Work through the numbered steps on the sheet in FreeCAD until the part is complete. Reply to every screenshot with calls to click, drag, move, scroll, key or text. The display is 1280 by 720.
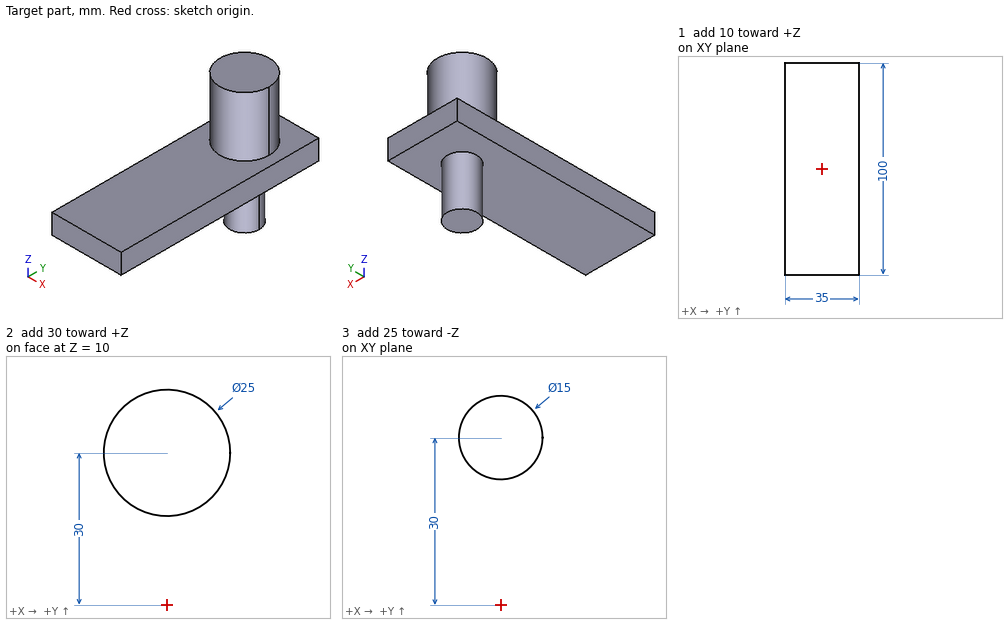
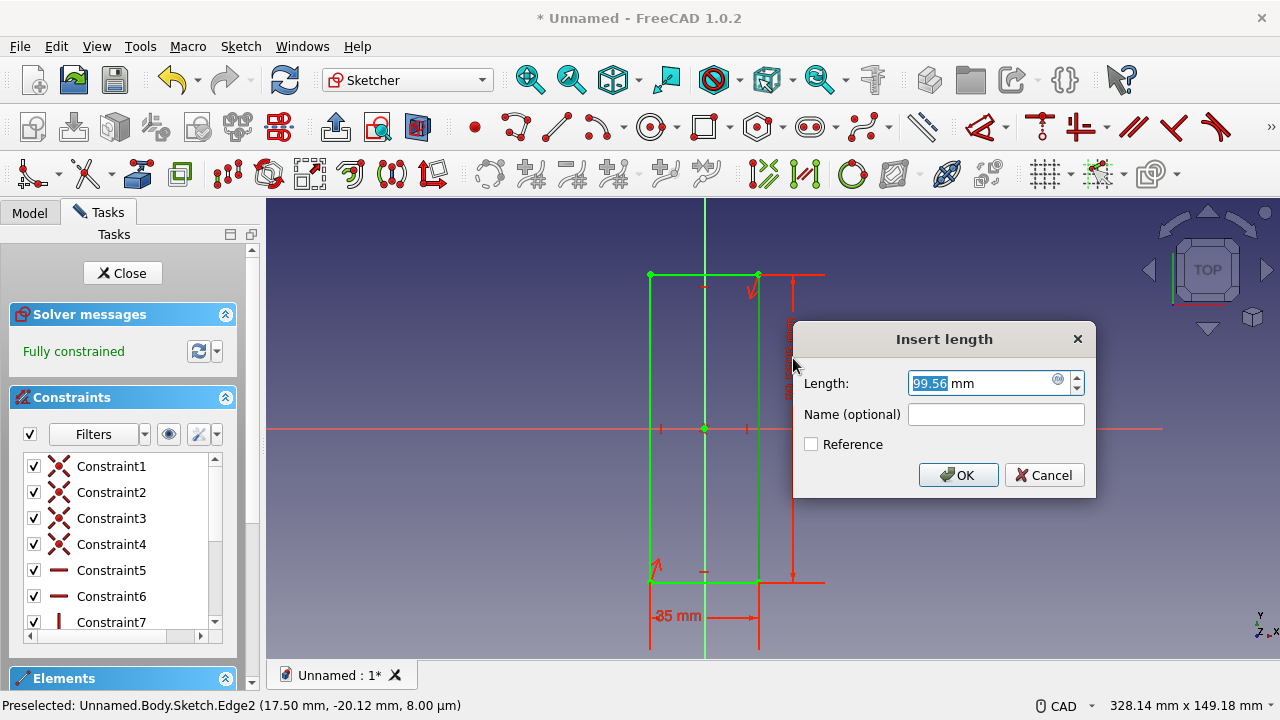
text(100)
key(Return)
key(Escape)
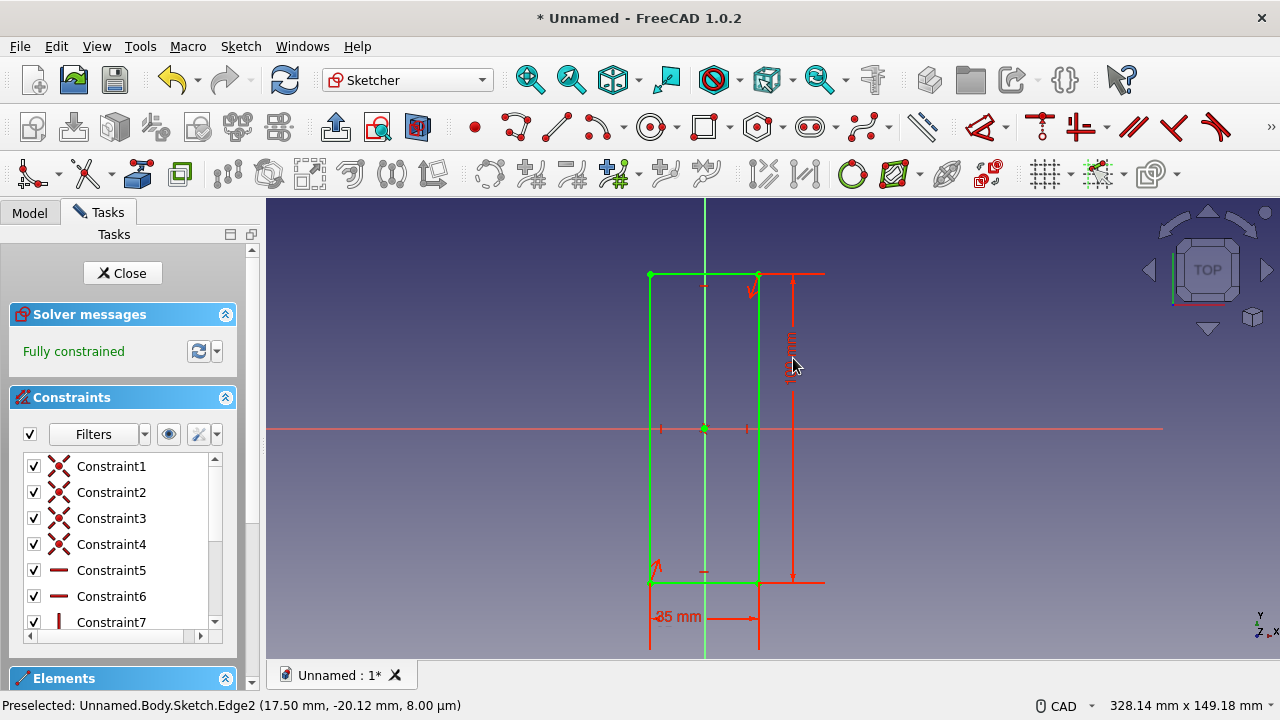
click(123, 273)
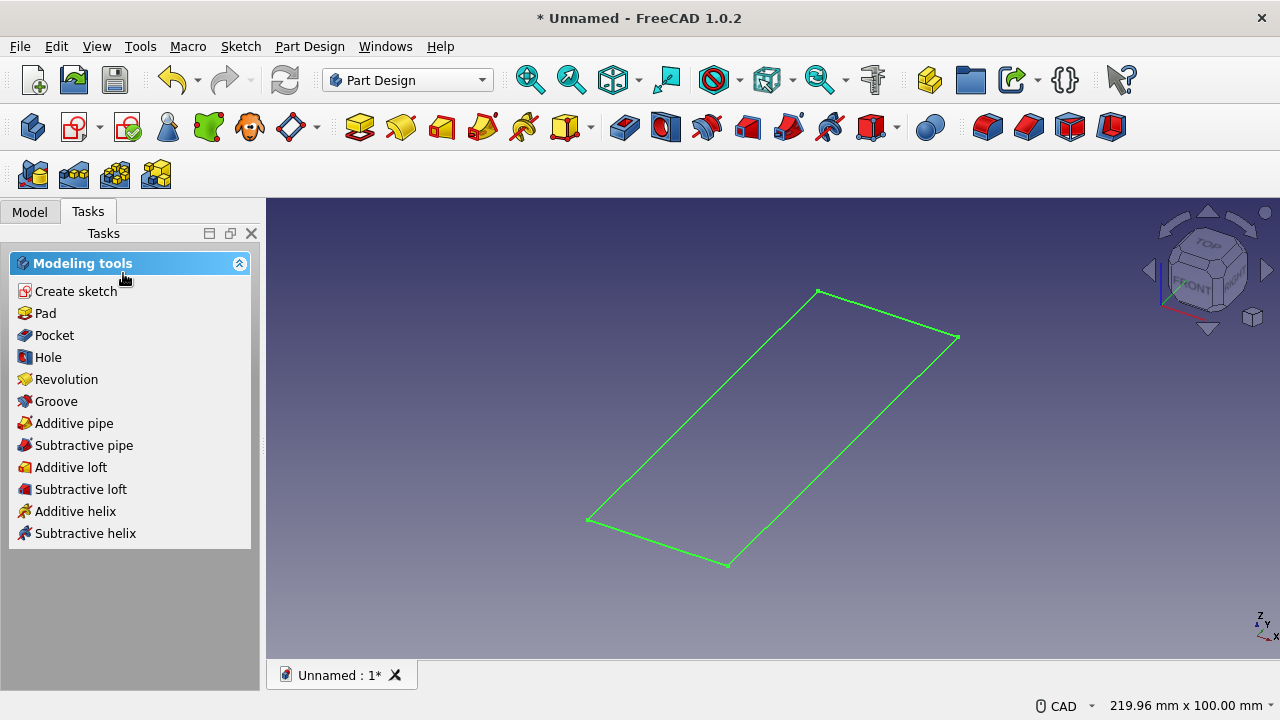
click(360, 128)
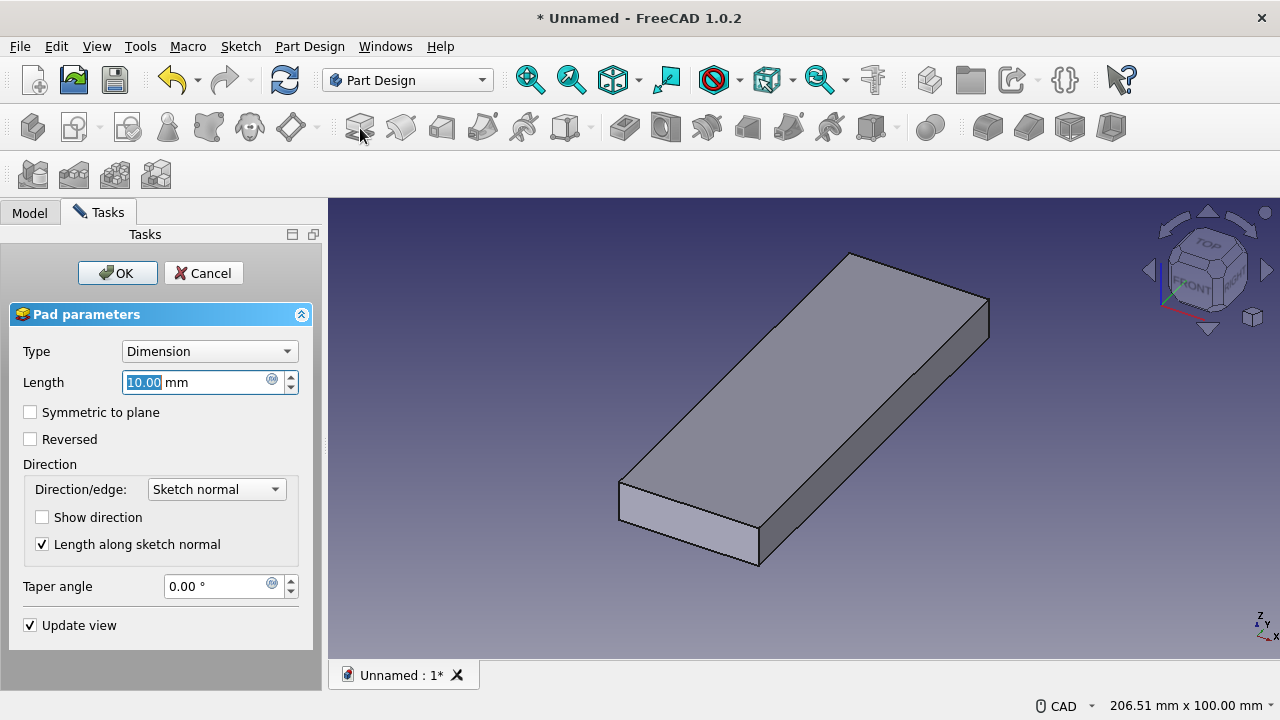
text(10)
key(Tab)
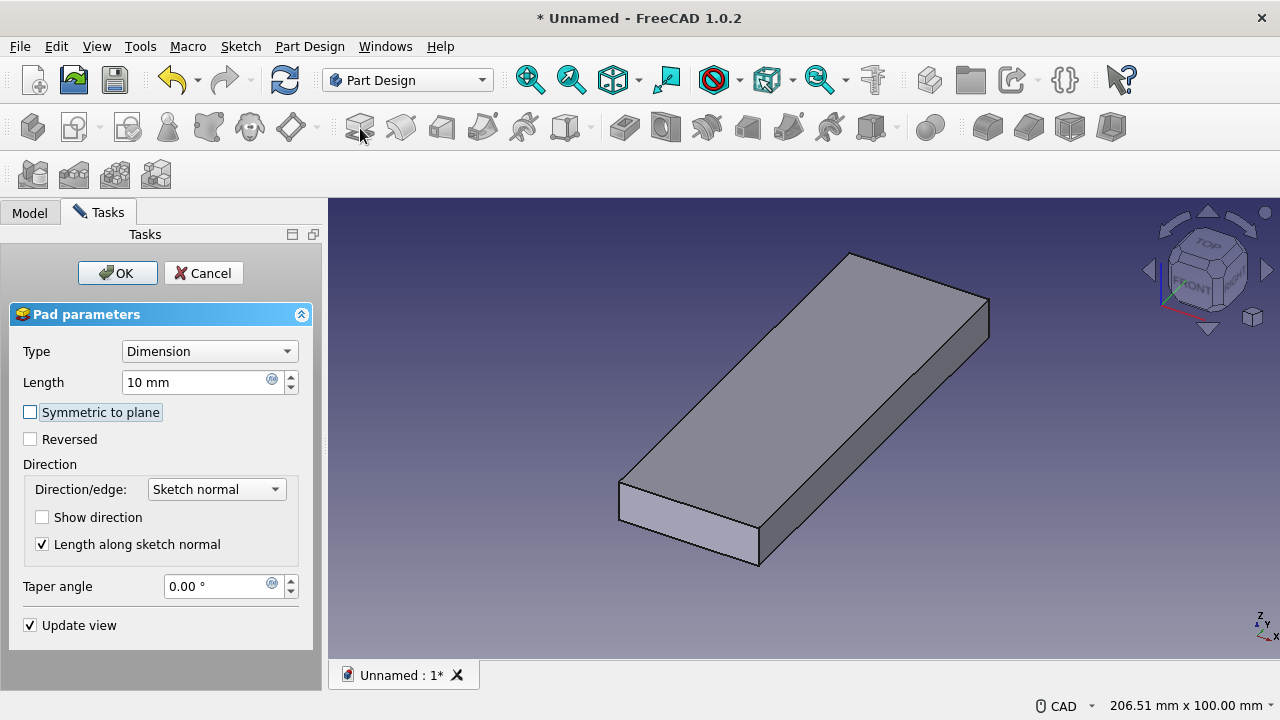
click(118, 273)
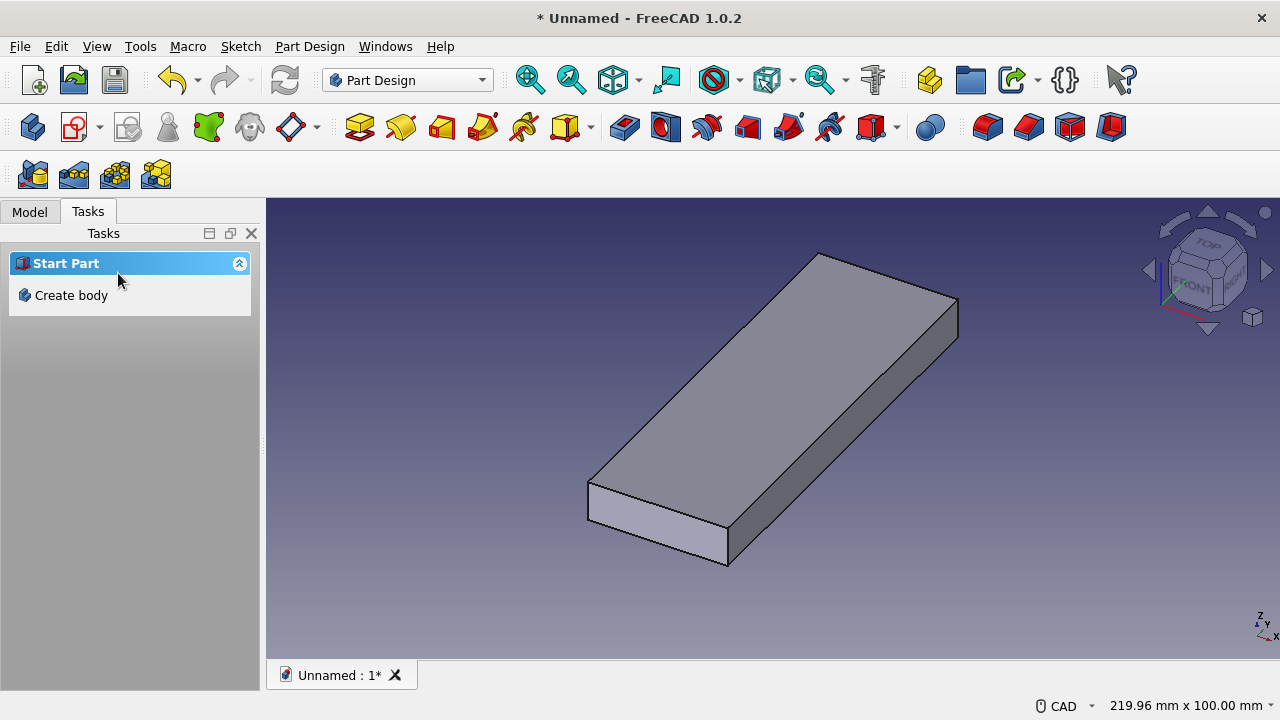
click(839, 324)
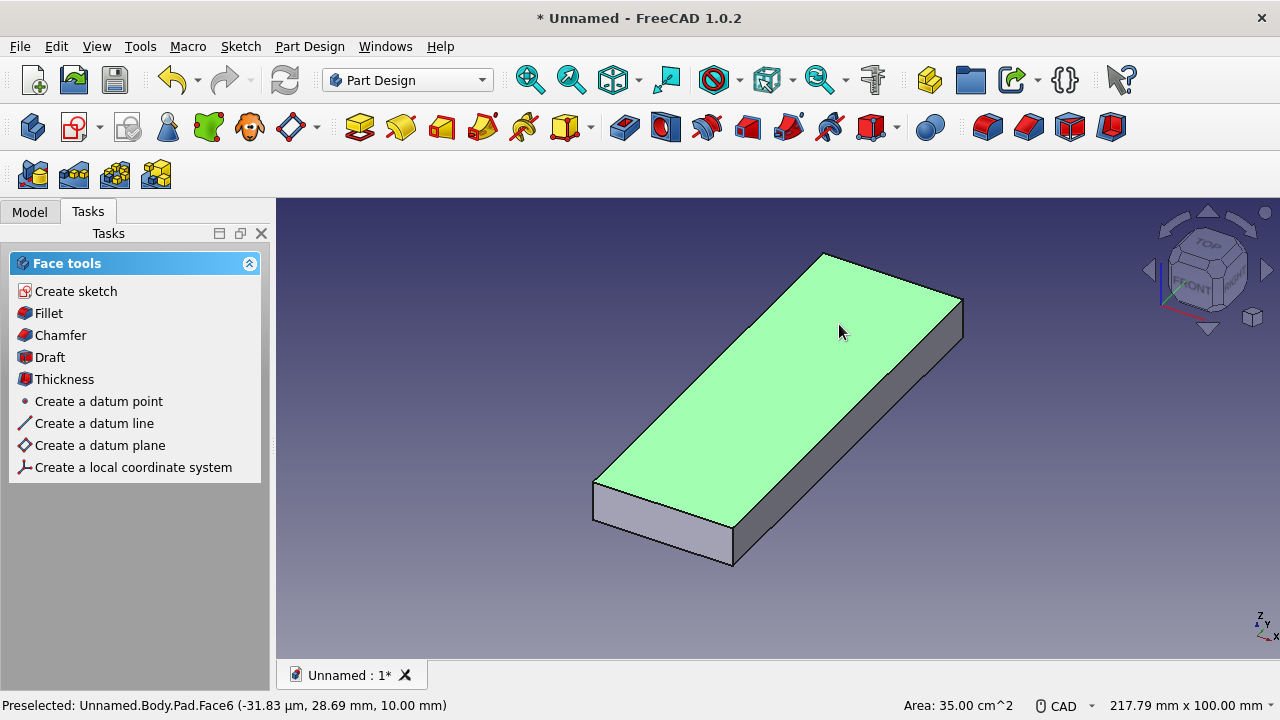
click(74, 128)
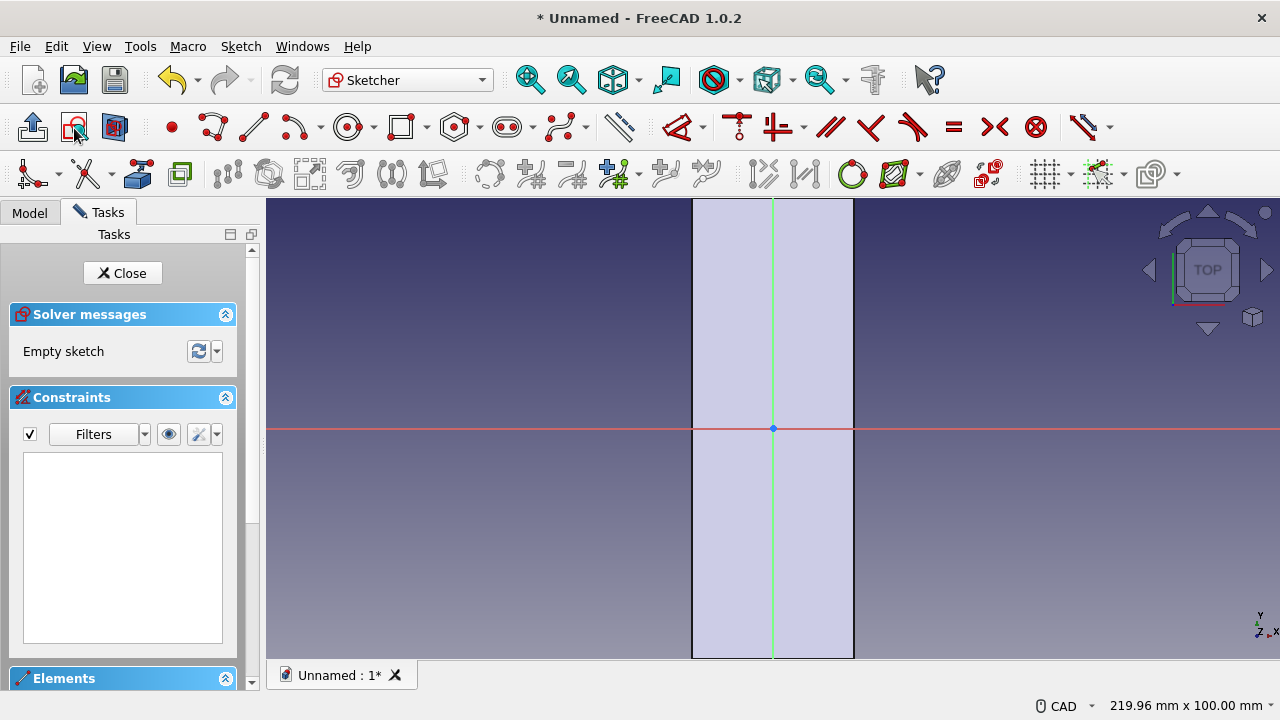
scroll(395, 631, down, 1)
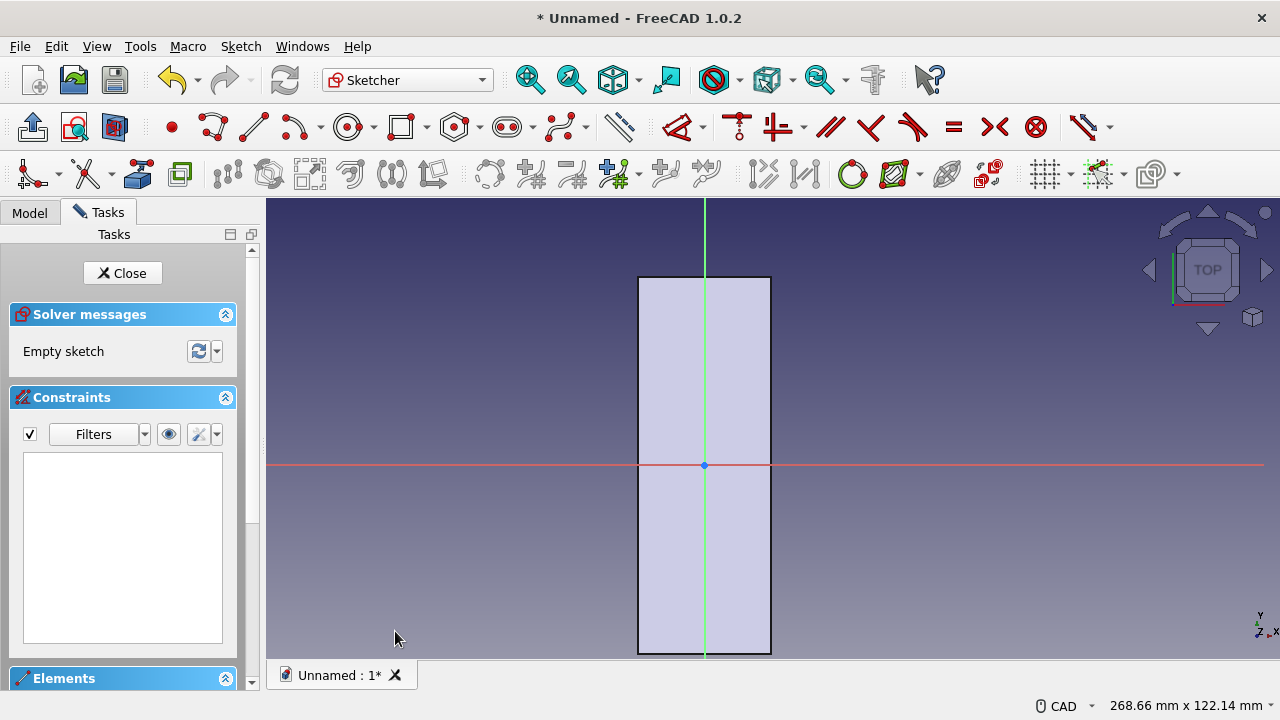
scroll(705, 332, up, 3)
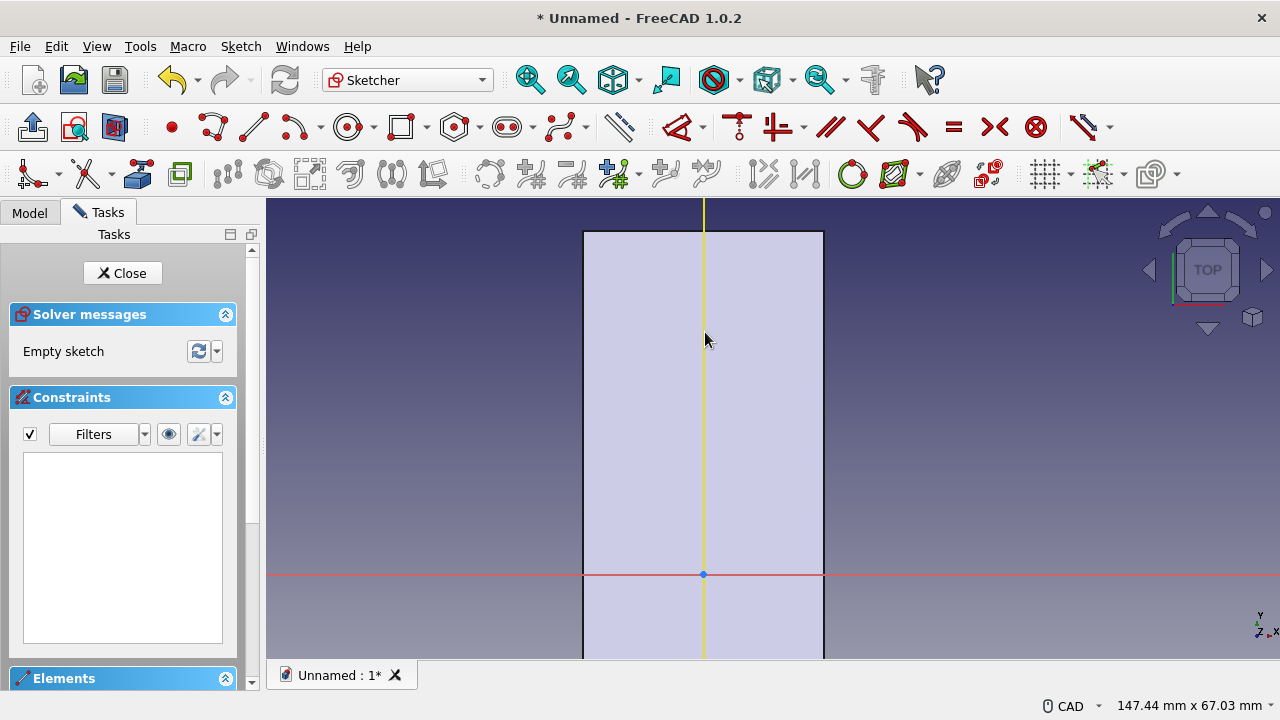
key(g)
key(c)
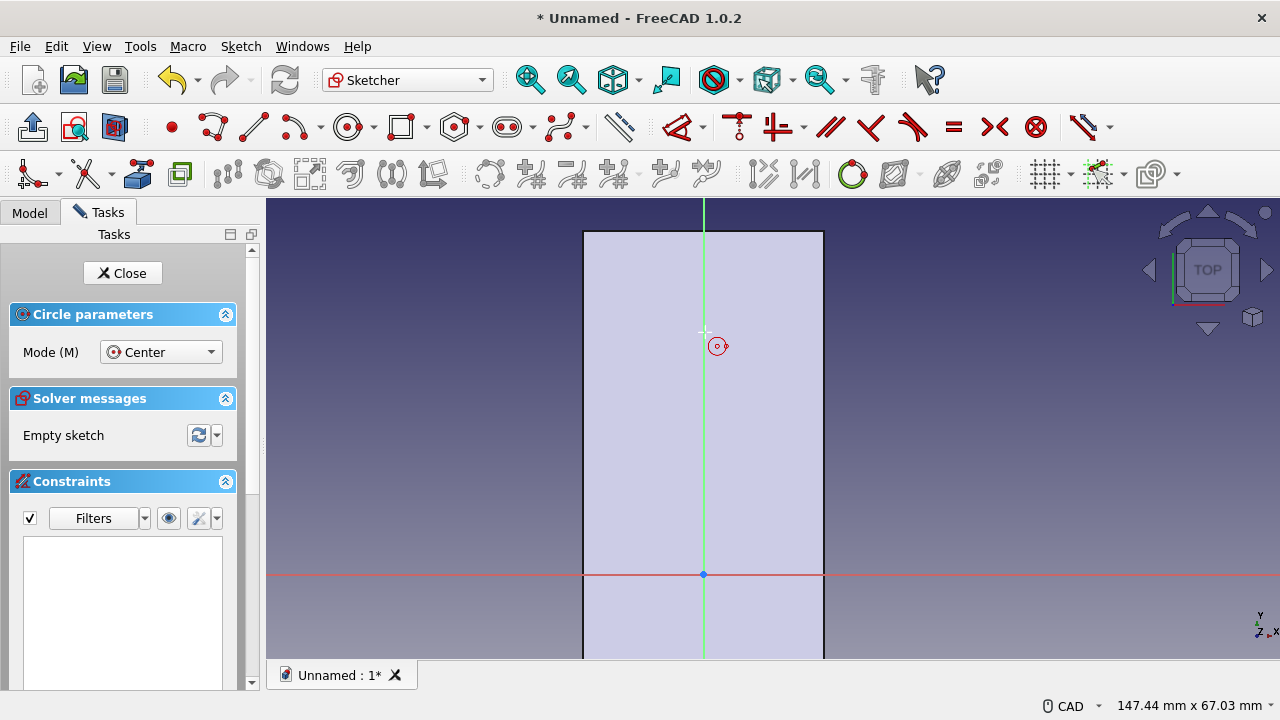
click(704, 368)
click(765, 308)
key(Escape)